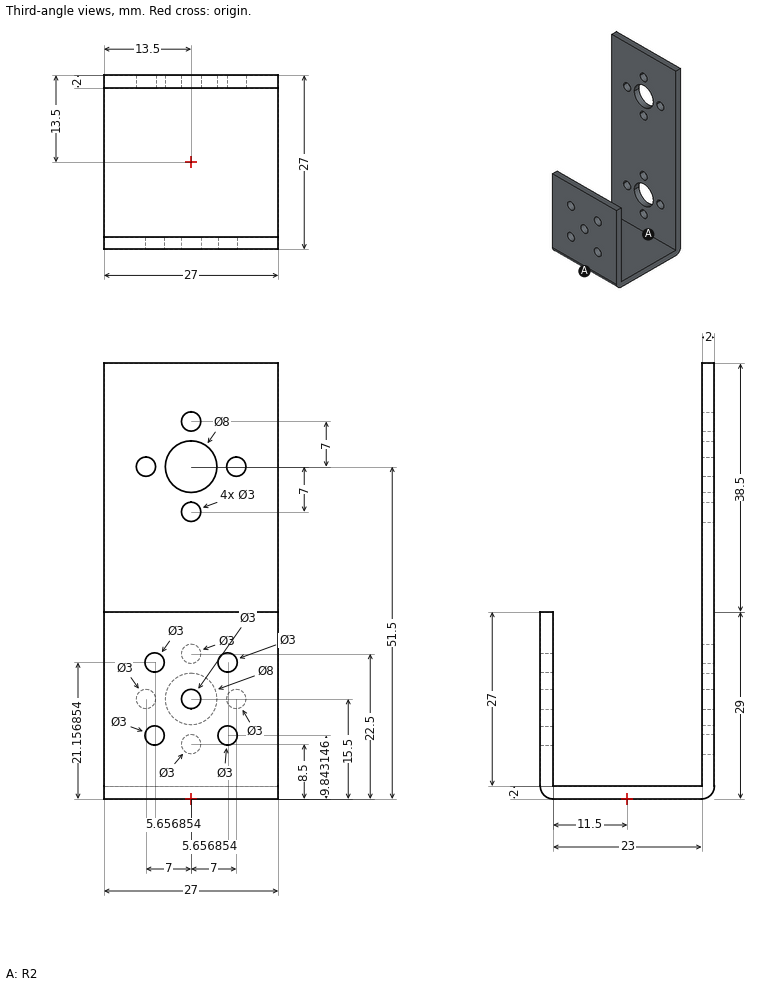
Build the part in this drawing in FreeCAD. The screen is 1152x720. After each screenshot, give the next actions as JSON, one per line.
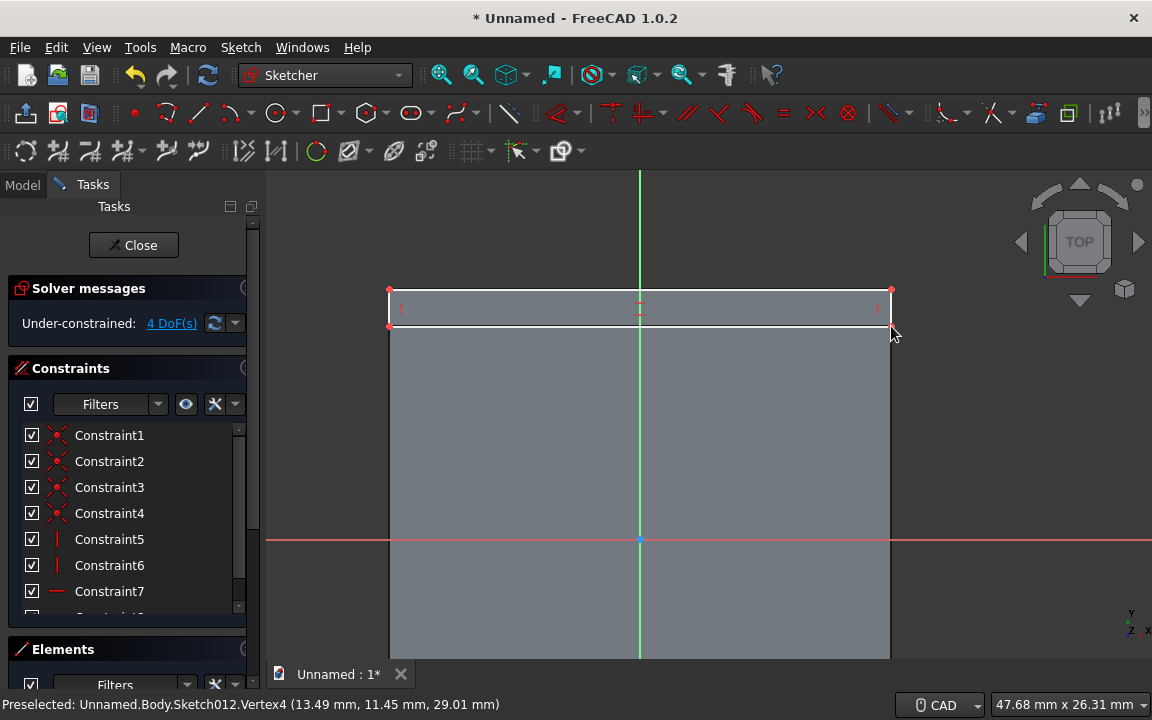
{"action": "key", "text": "d"}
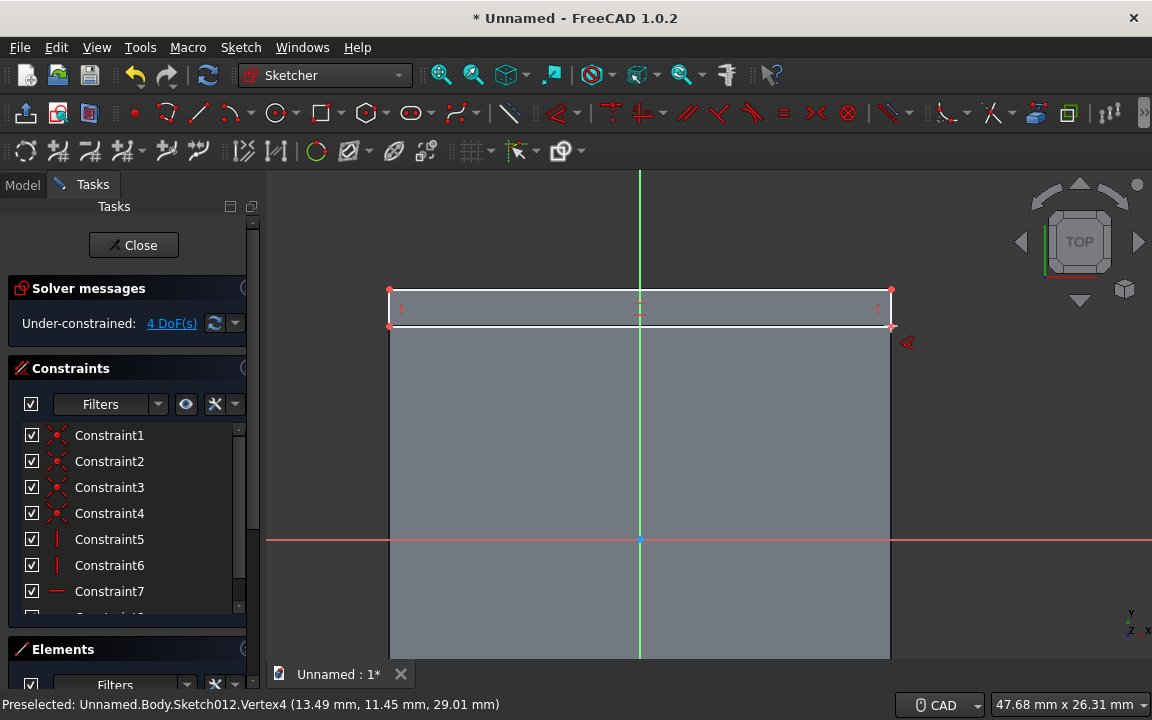
{"action": "scroll", "coordinate": [389, 301], "scroll_direction": "up", "scroll_amount": 2}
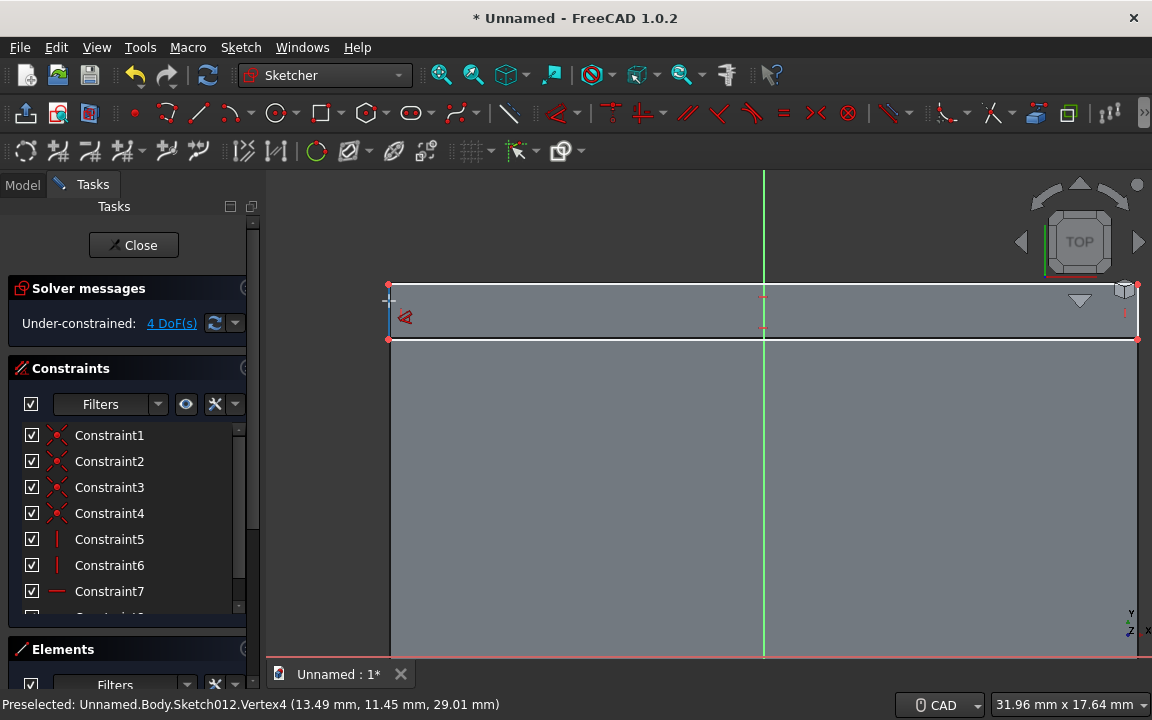
{"action": "left_click", "coordinate": [389, 301]}
{"action": "left_click", "coordinate": [355, 312]}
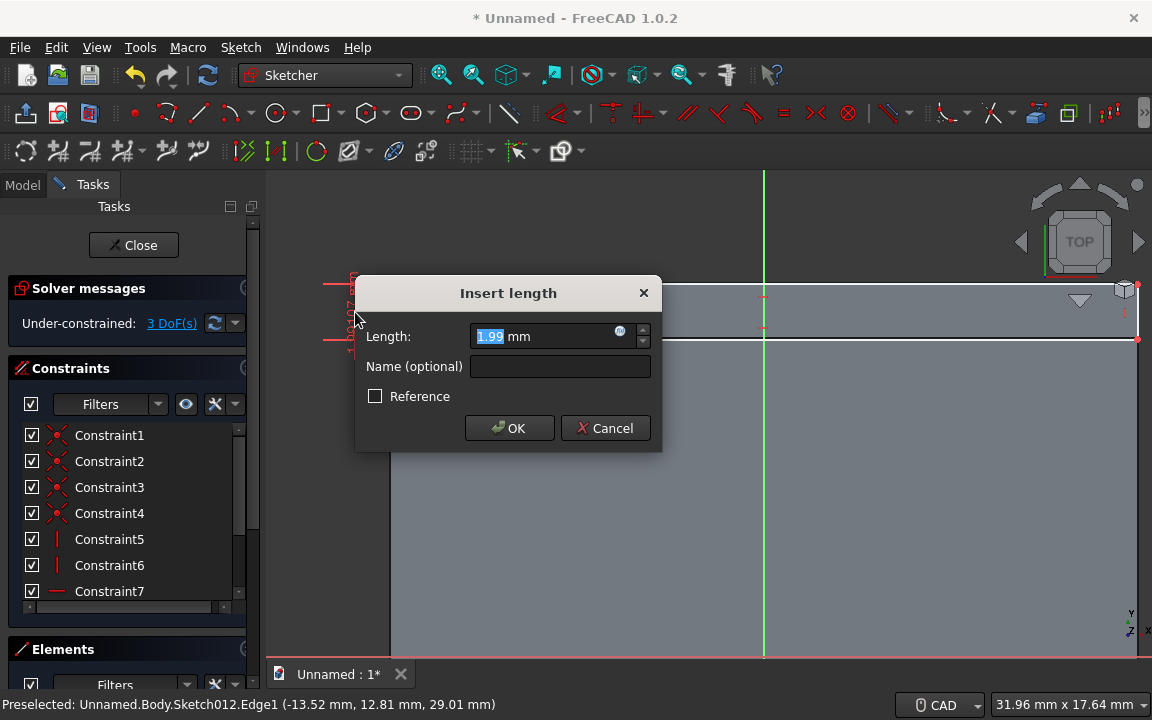
{"action": "type", "text": "2"}
{"action": "key", "text": "Return"}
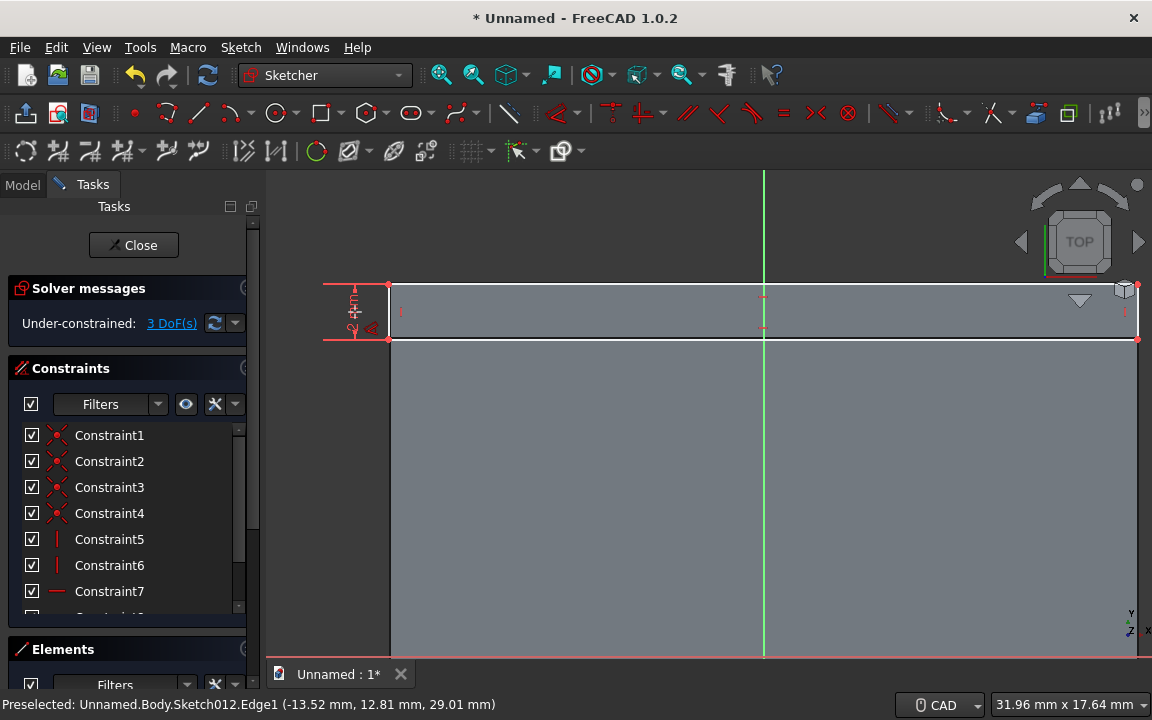
{"action": "left_click", "coordinate": [614, 340]}
{"action": "left_click", "coordinate": [688, 306]}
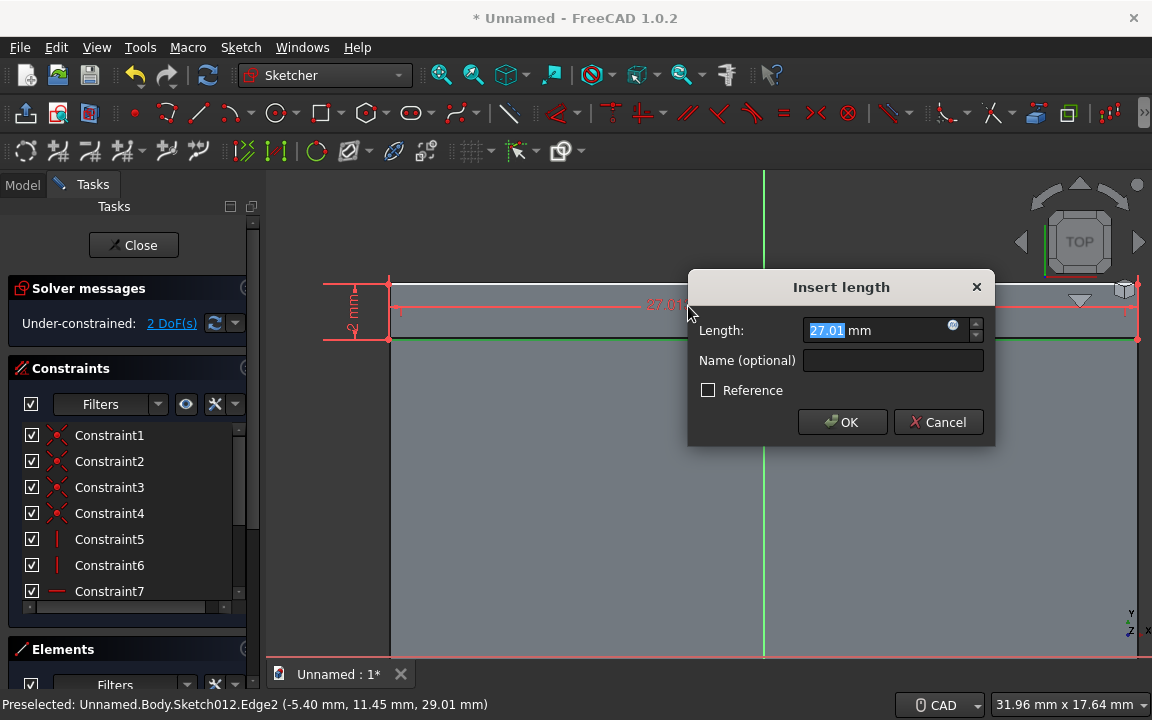
{"action": "type", "text": "27"}
{"action": "key", "text": "Return"}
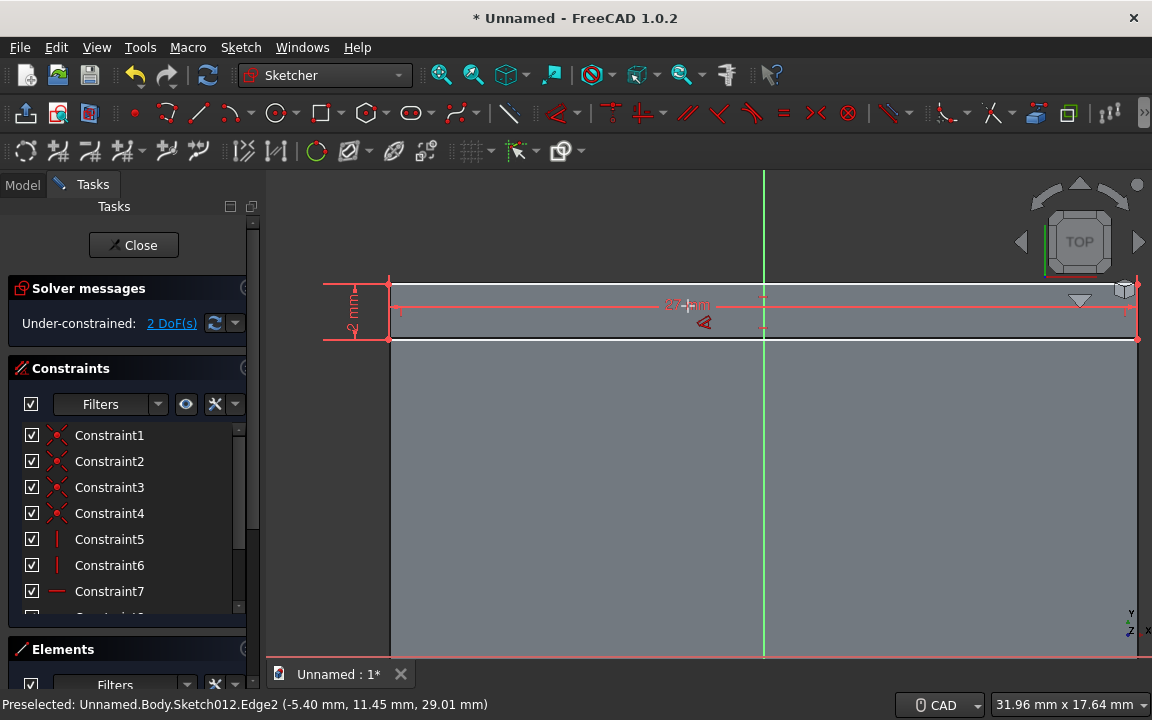
{"action": "left_click", "coordinate": [389, 284]}
{"action": "left_click", "coordinate": [576, 250]}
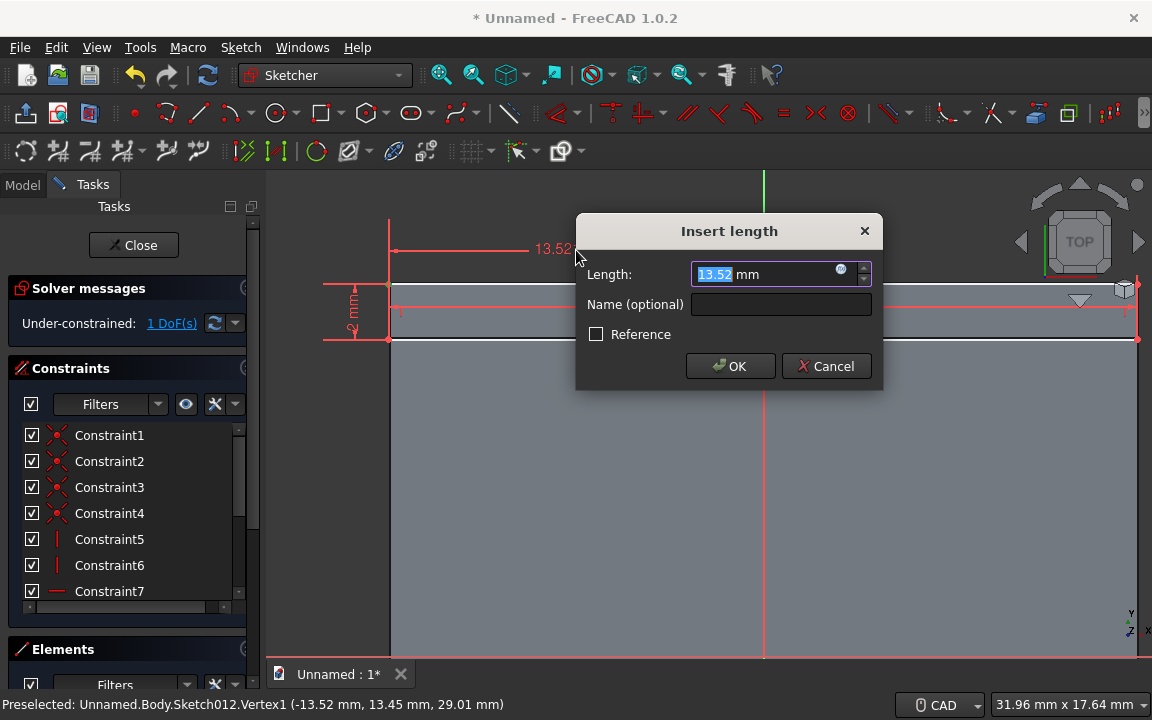
{"action": "type", "text": "13.5"}
{"action": "key", "text": "Return"}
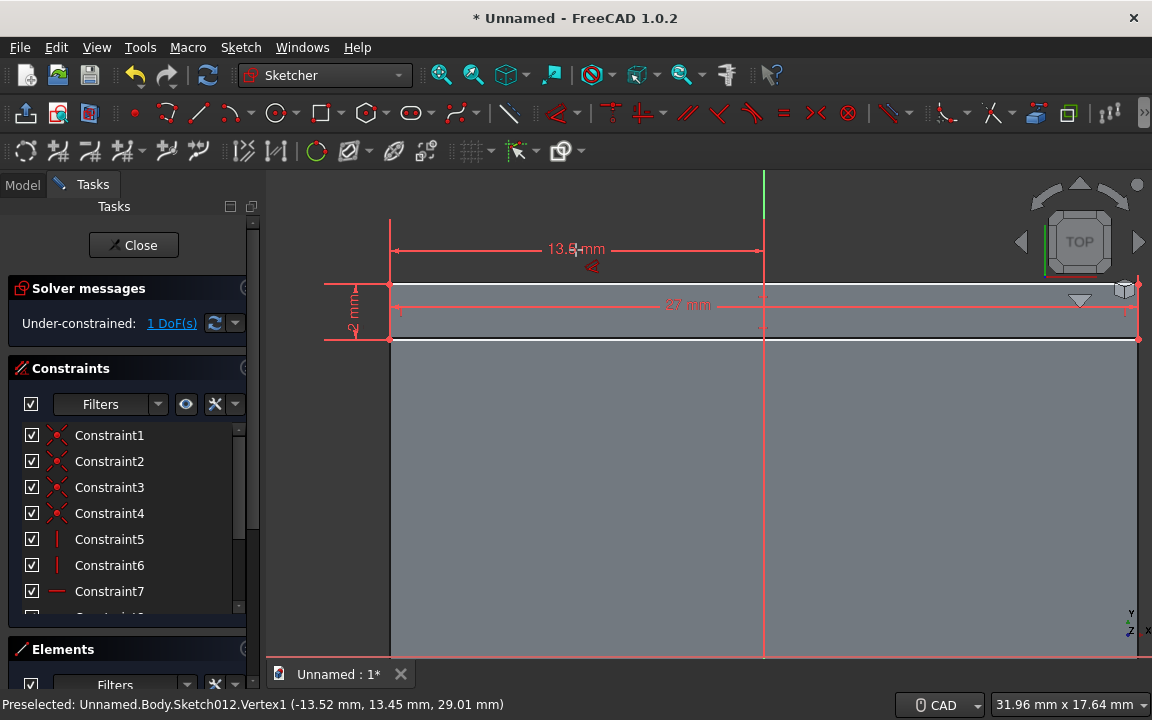
{"action": "left_click", "coordinate": [390, 284]}
{"action": "left_click", "coordinate": [356, 458]}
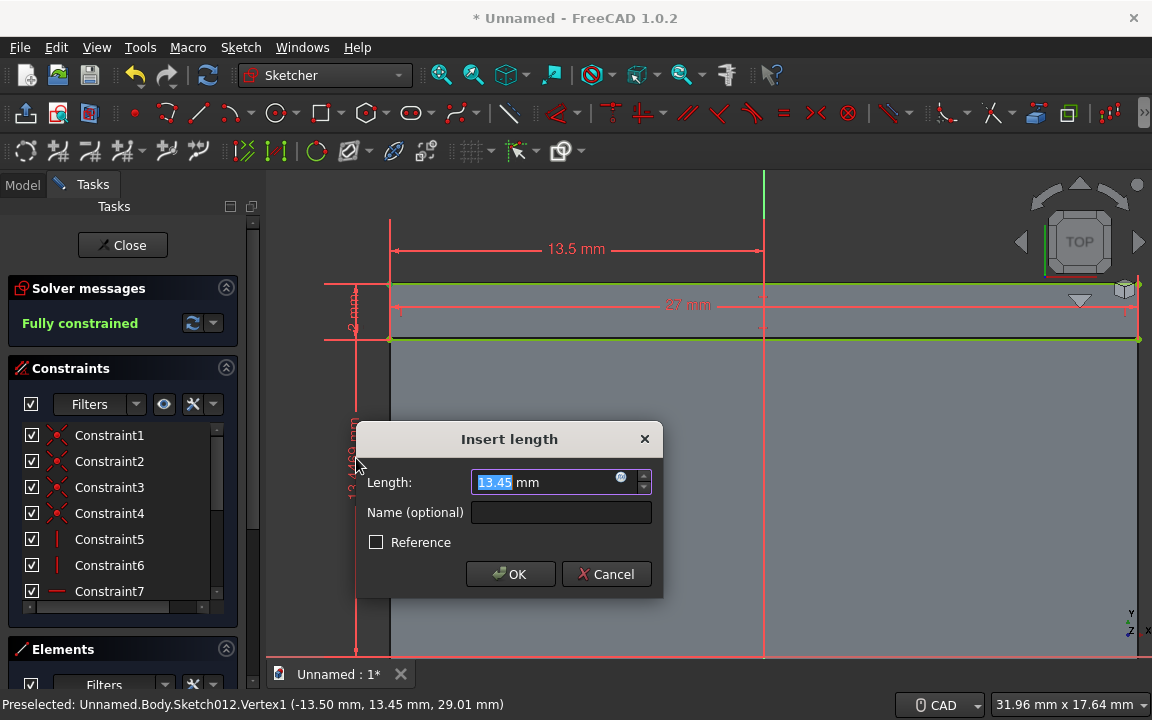
{"action": "type", "text": "13.5"}
{"action": "key", "text": "Return"}
{"action": "key", "text": "Escape"}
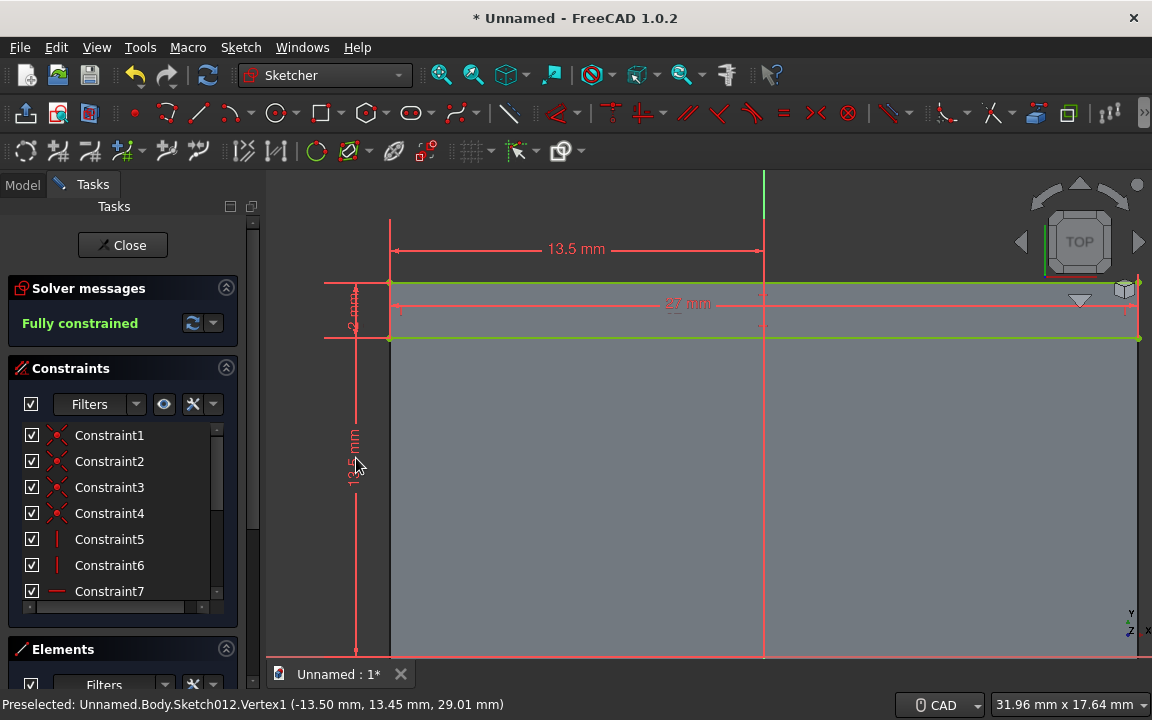
{"action": "left_click", "coordinate": [123, 245]}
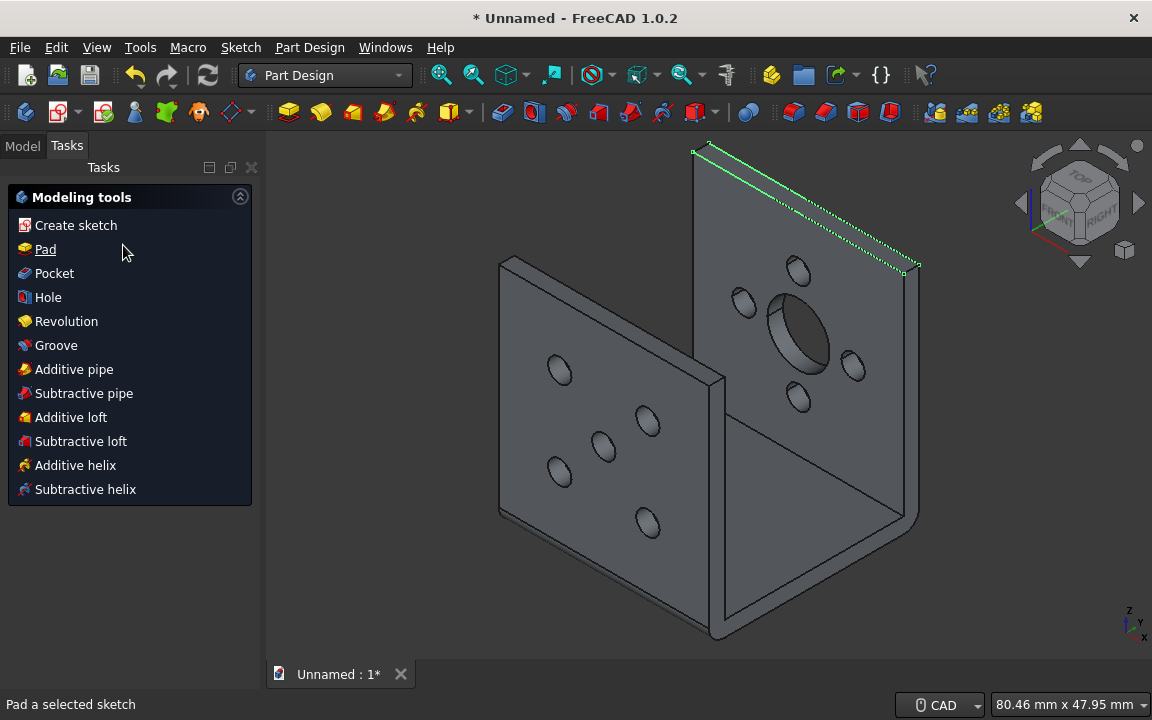
{"action": "left_click", "coordinate": [290, 112]}